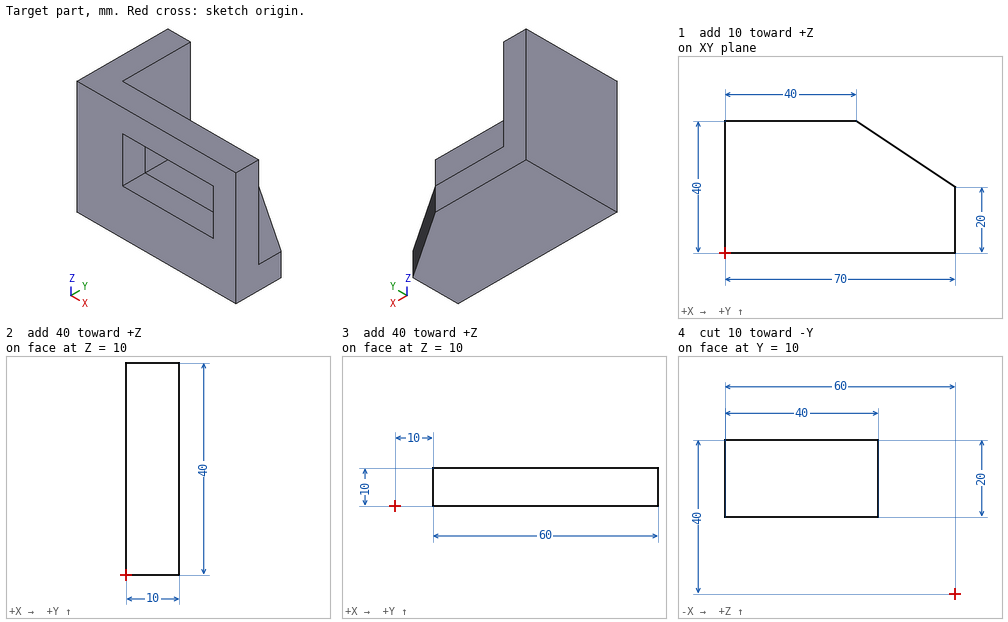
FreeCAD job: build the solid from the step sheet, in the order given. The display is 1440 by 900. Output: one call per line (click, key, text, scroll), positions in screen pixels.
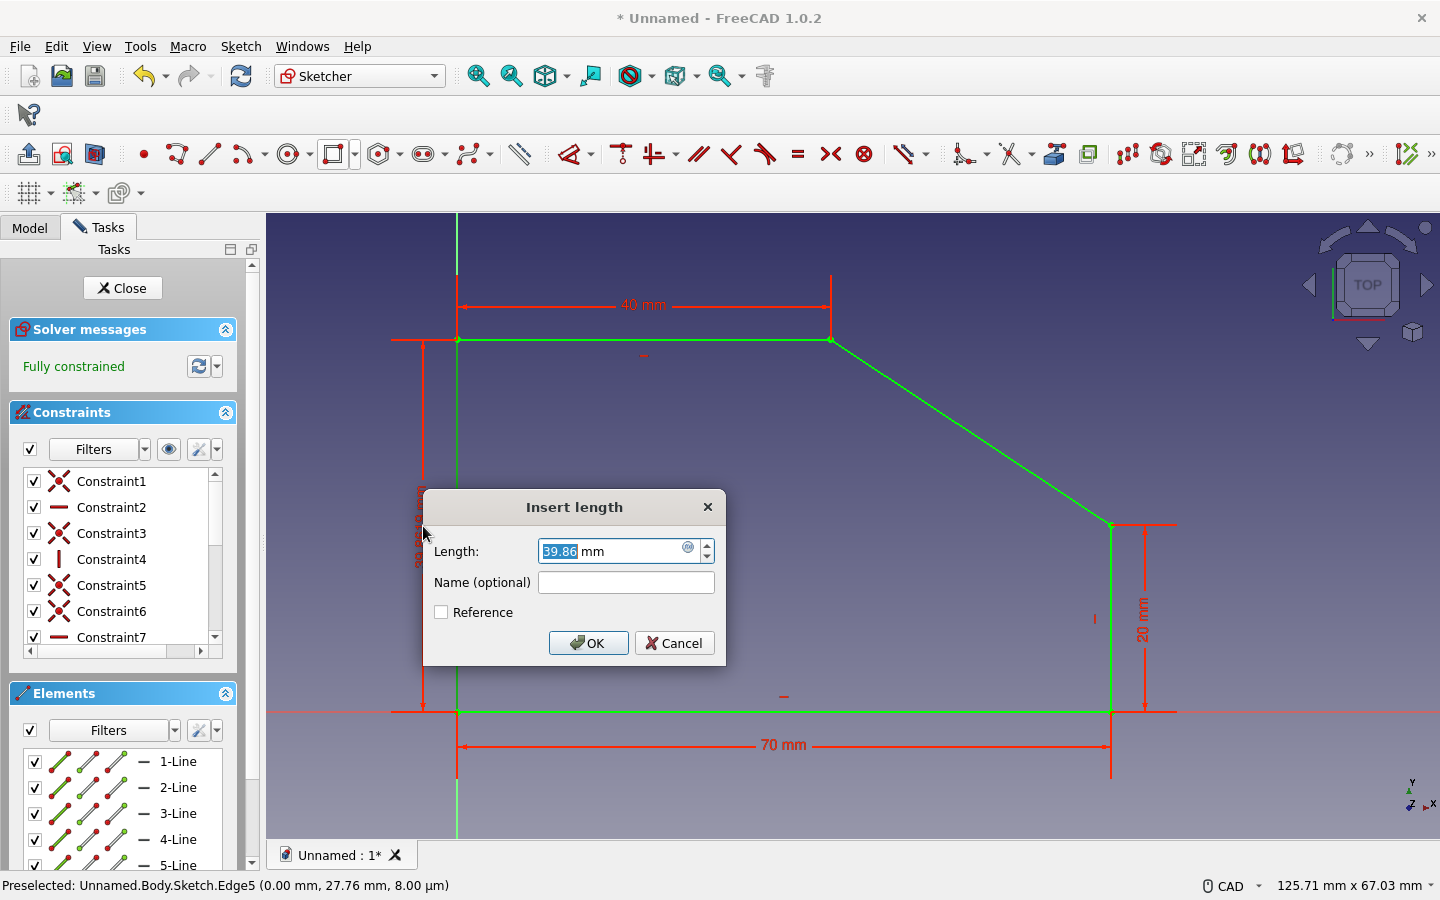
text(40)
key(Return)
key(Escape)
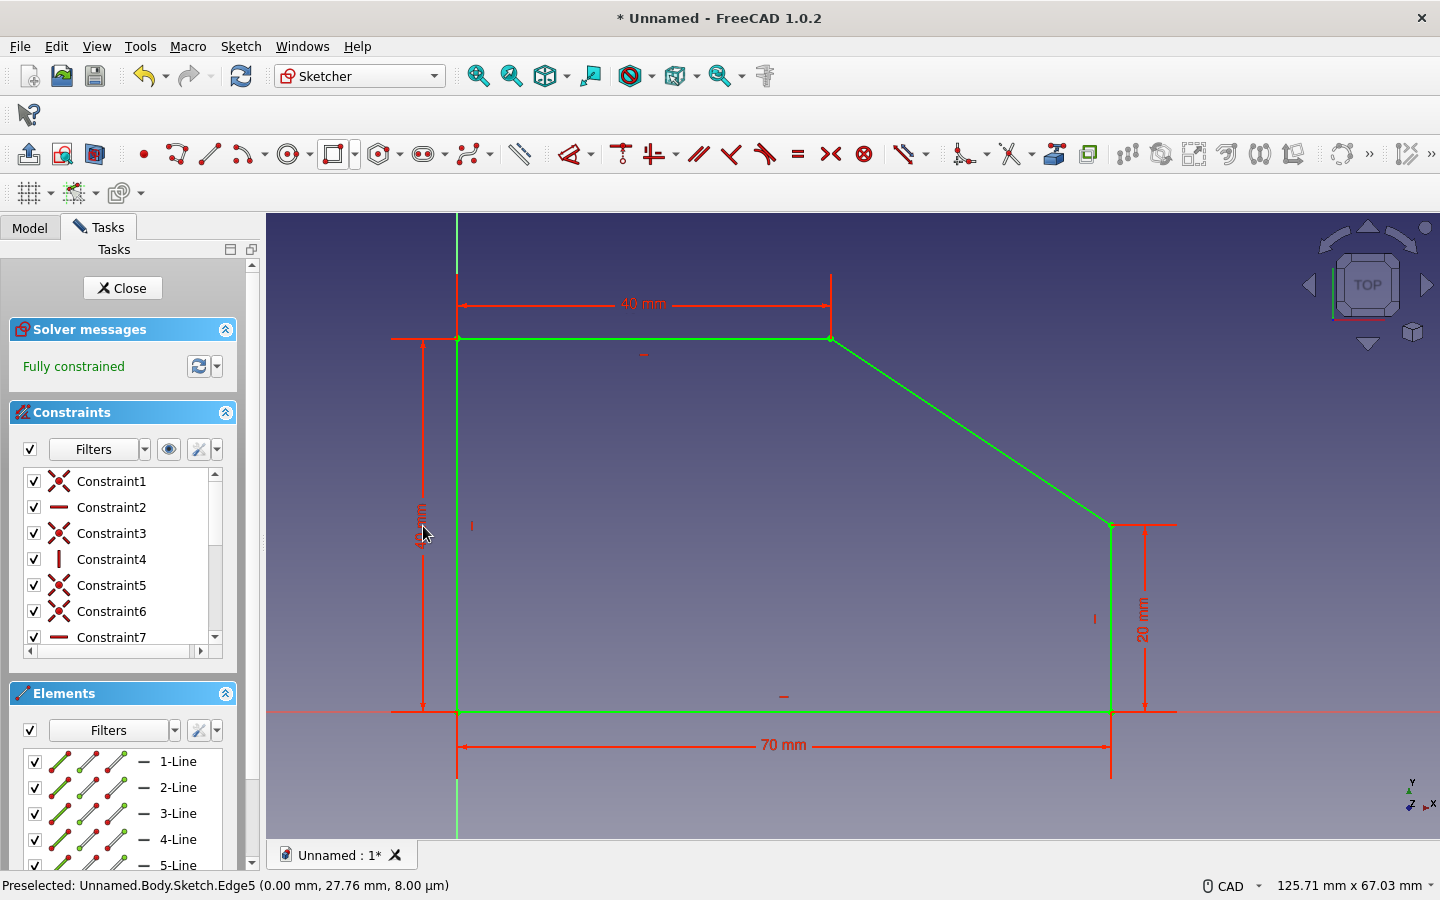
click(123, 288)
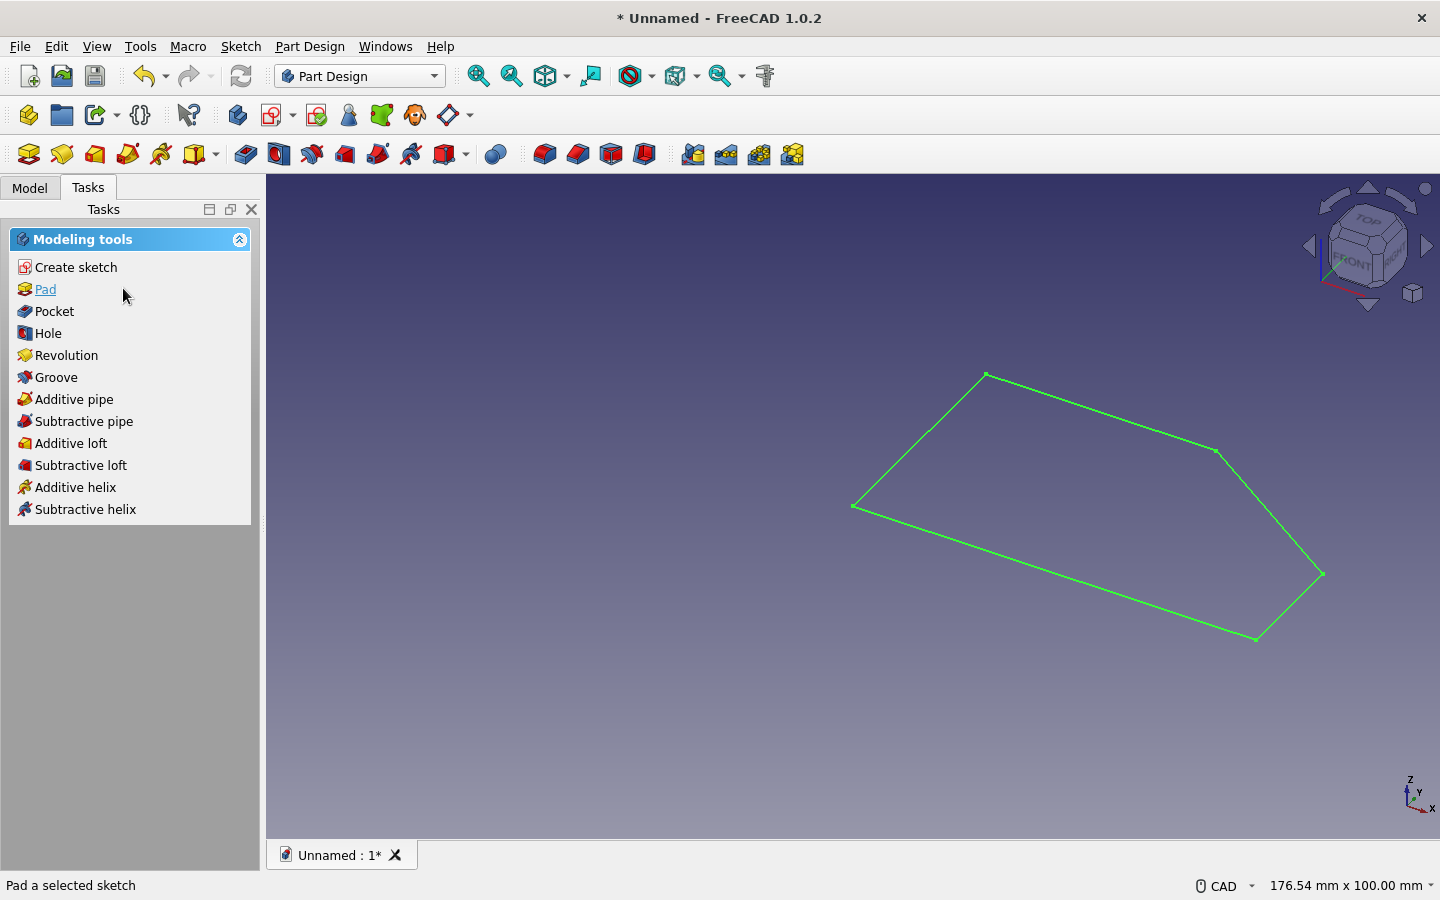
click(29, 154)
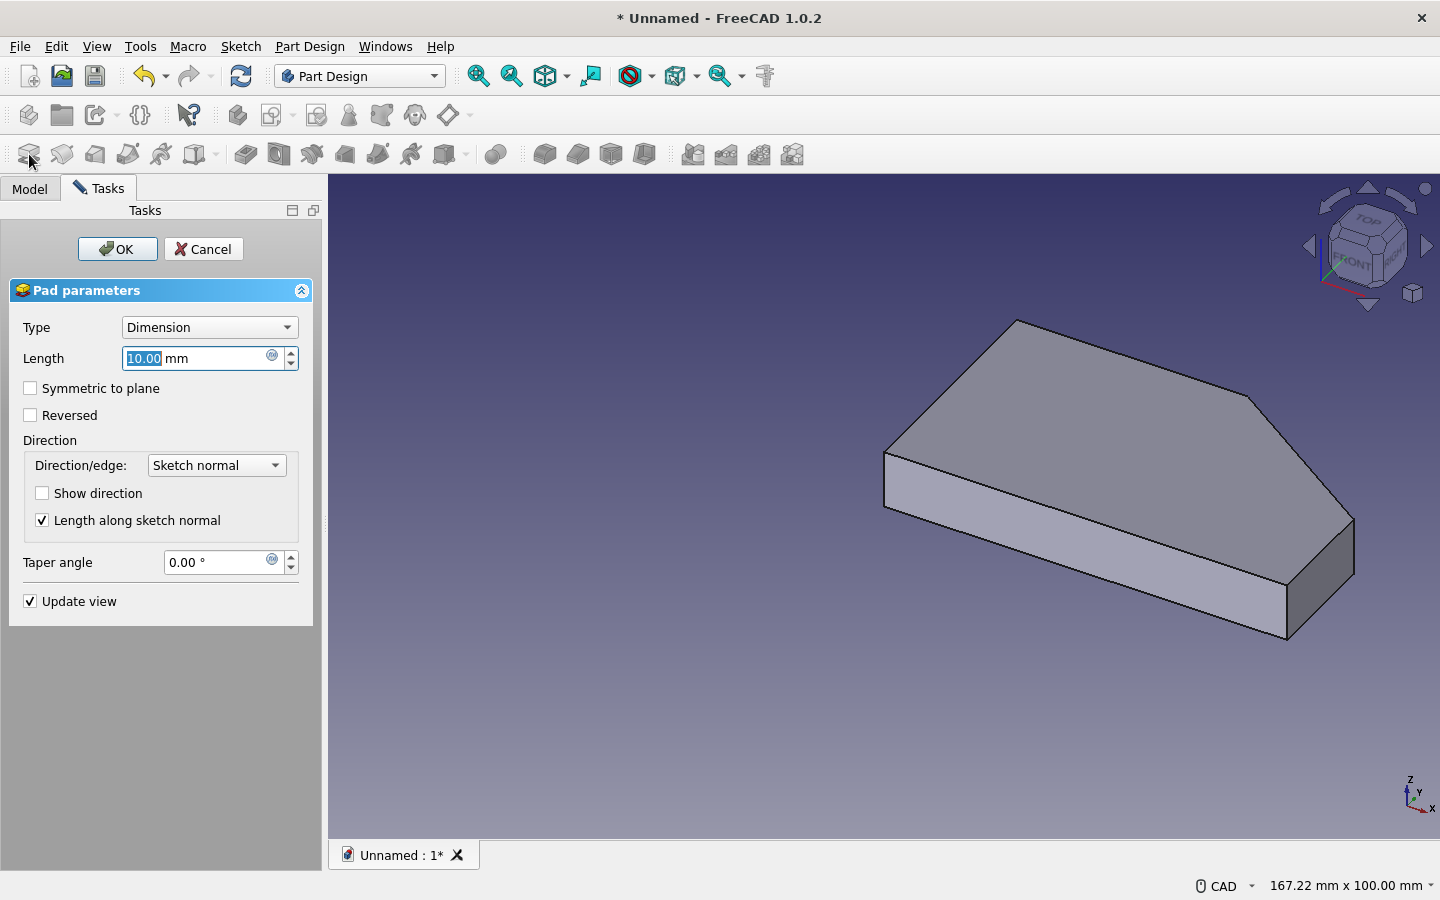
text(10)
key(Tab)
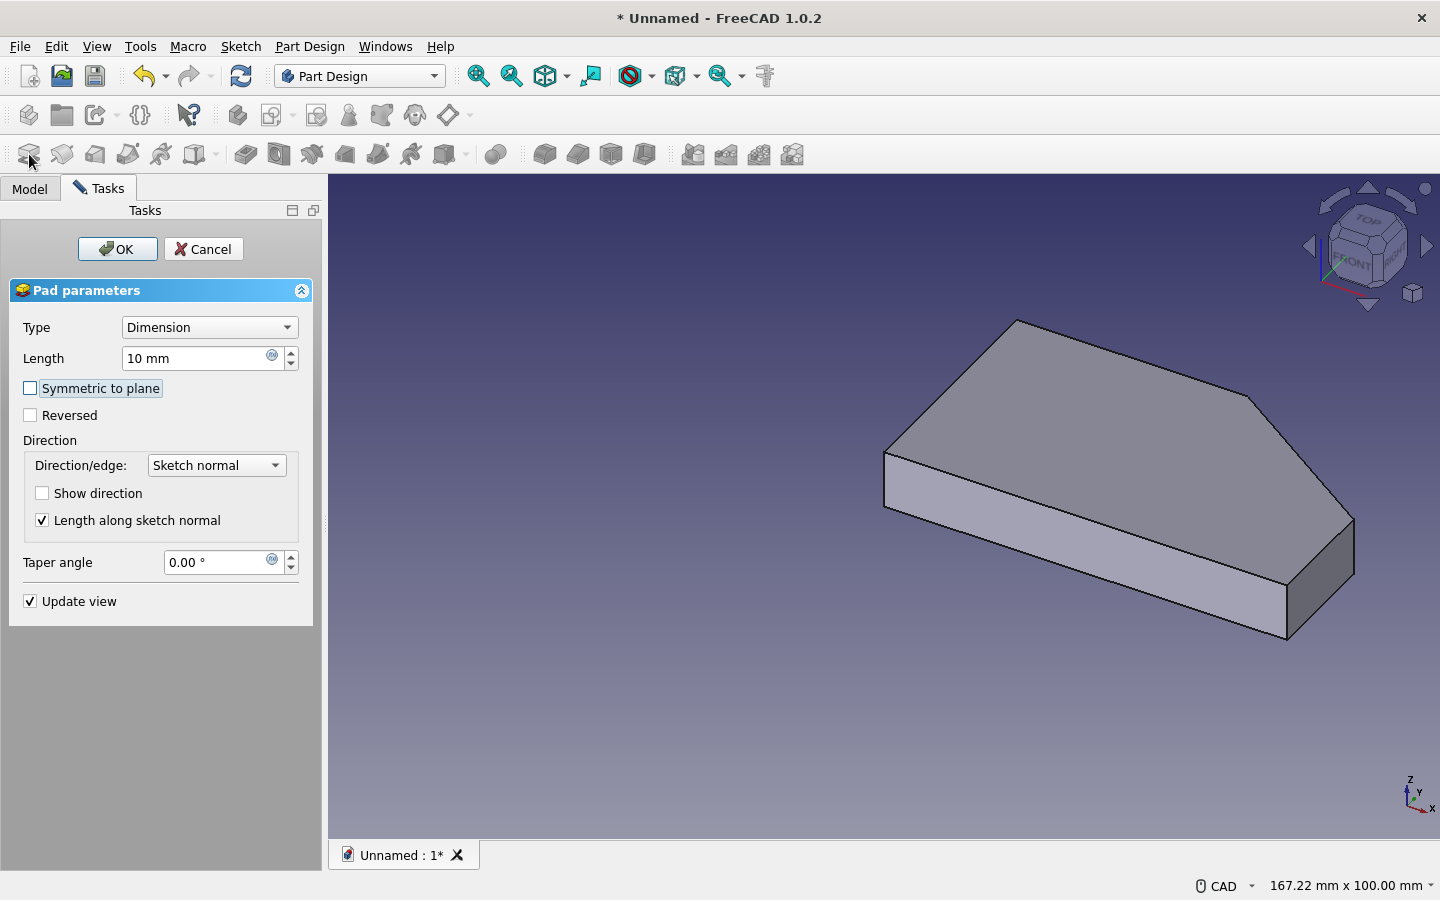
click(118, 249)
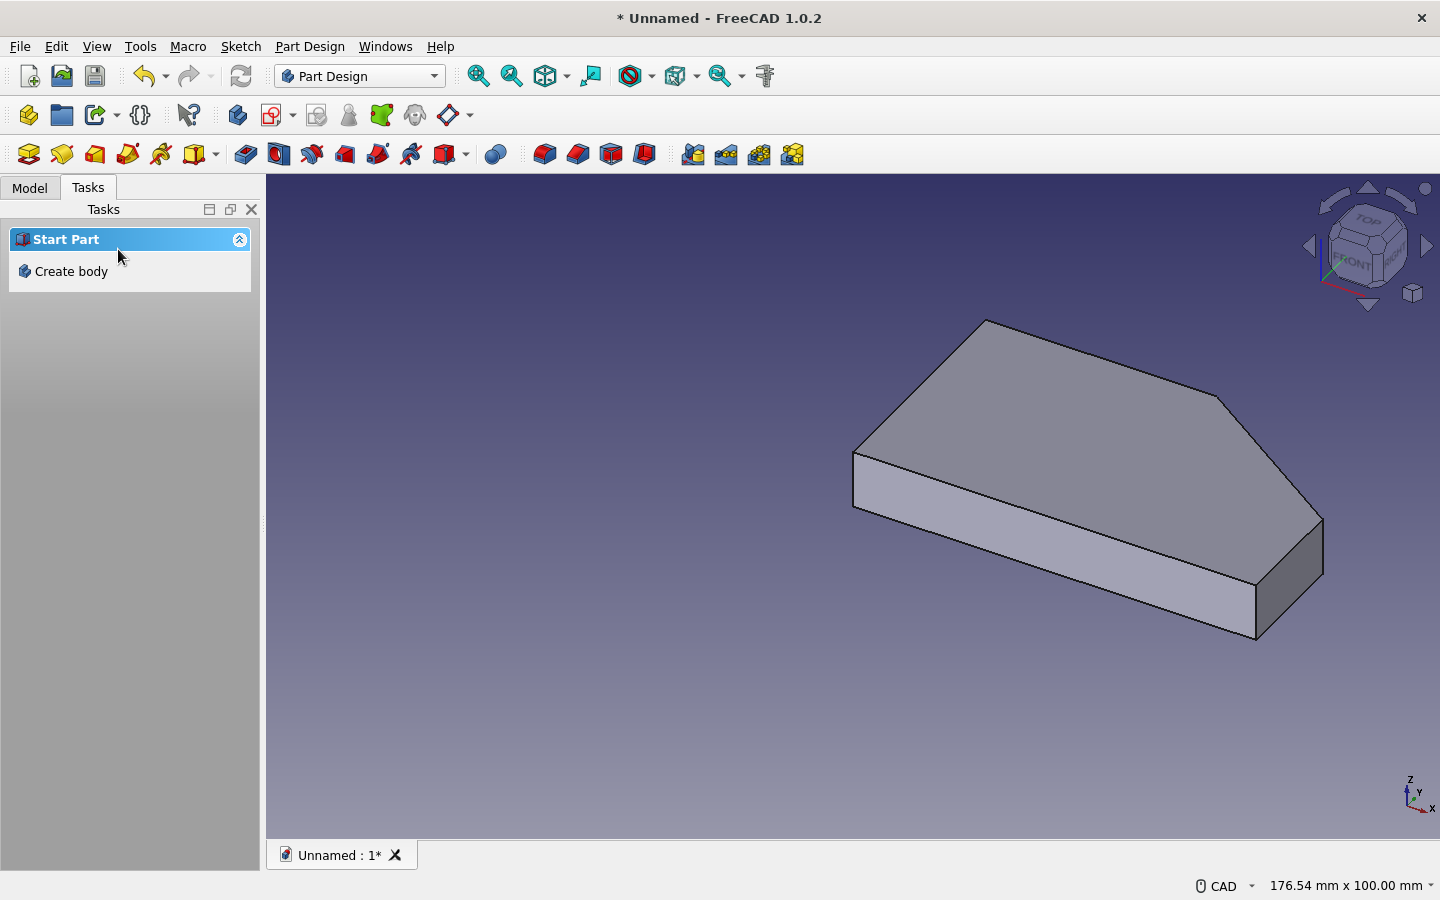
click(1063, 433)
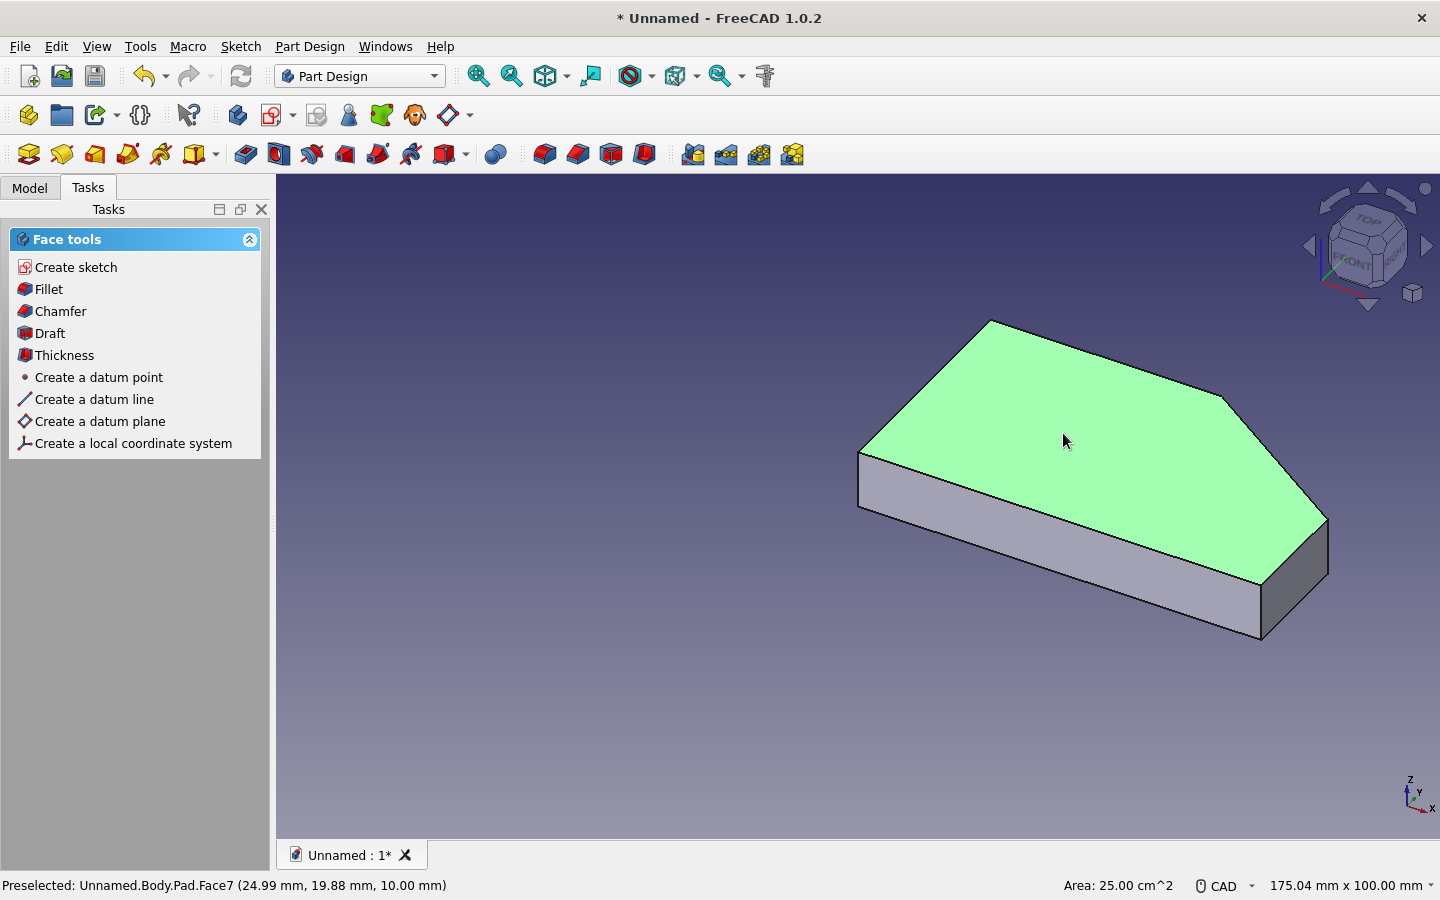
click(270, 116)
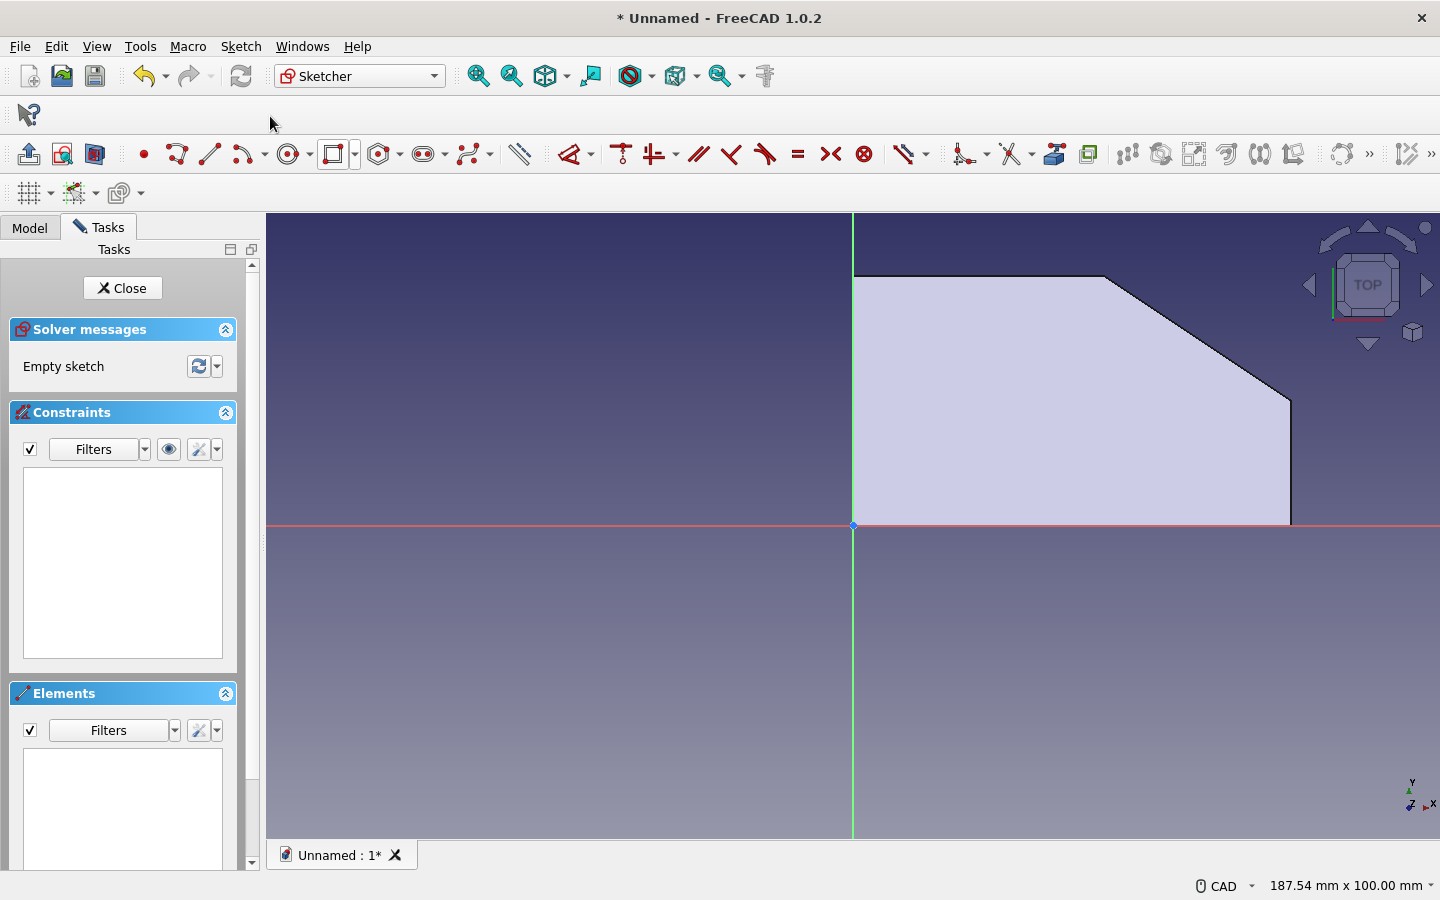
scroll(1087, 241, up, 2)